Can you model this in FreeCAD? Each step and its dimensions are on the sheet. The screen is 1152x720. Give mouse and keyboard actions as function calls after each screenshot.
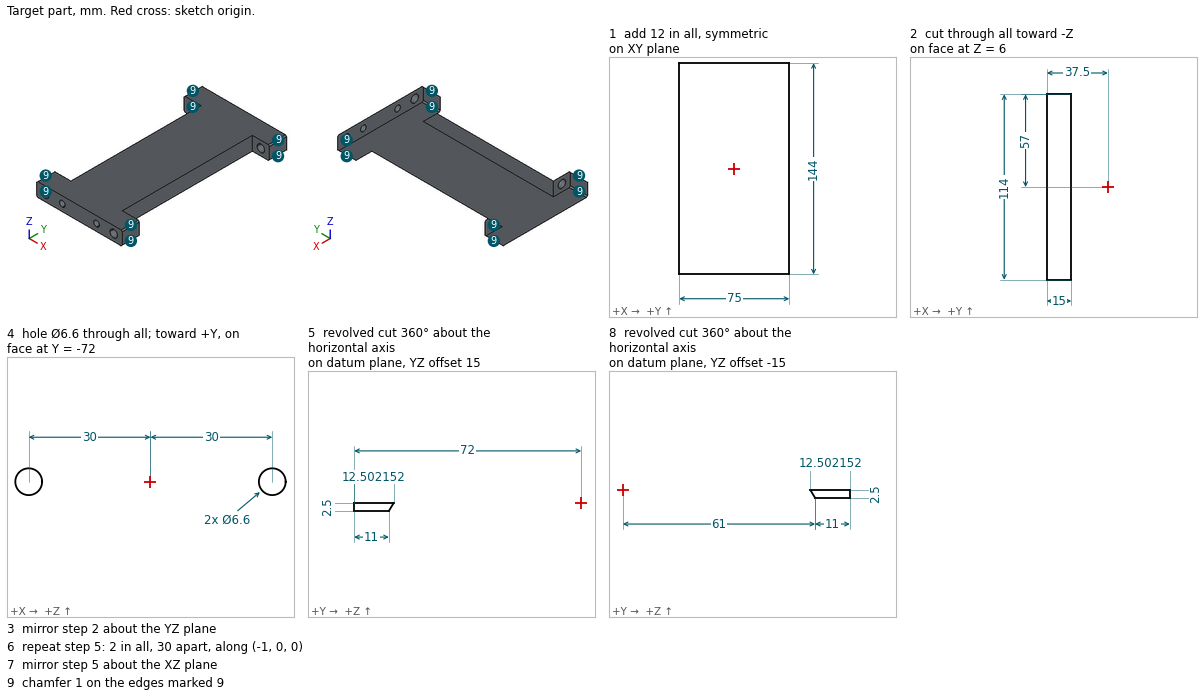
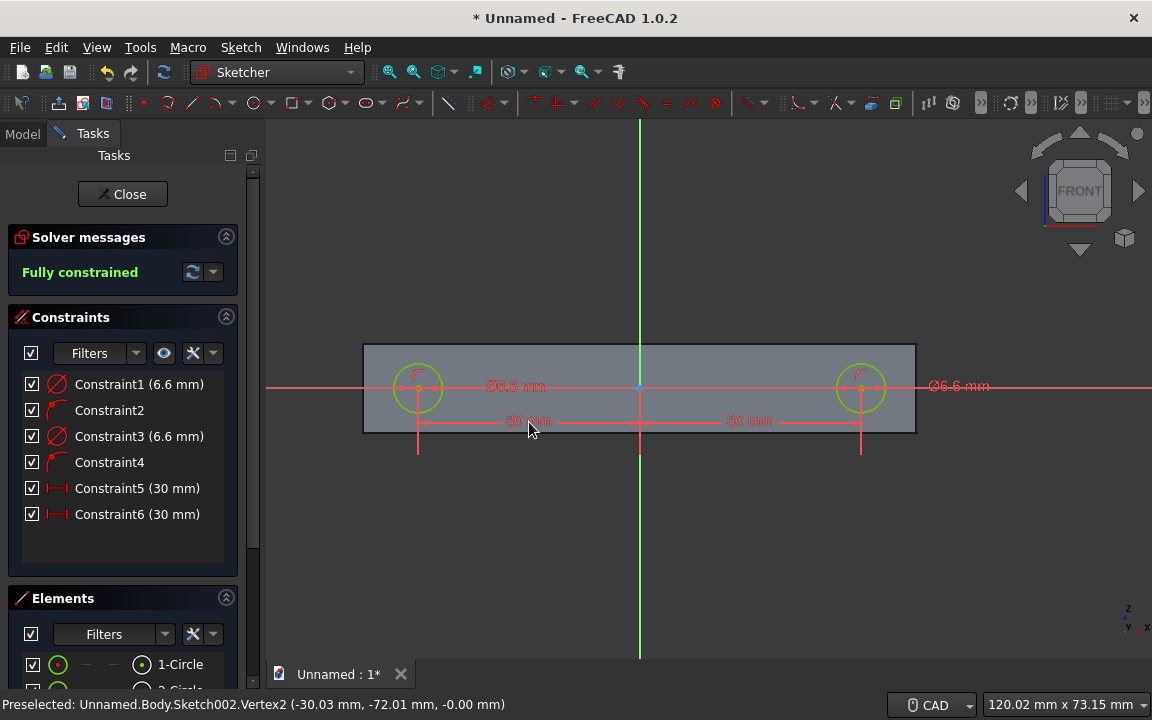
click(123, 194)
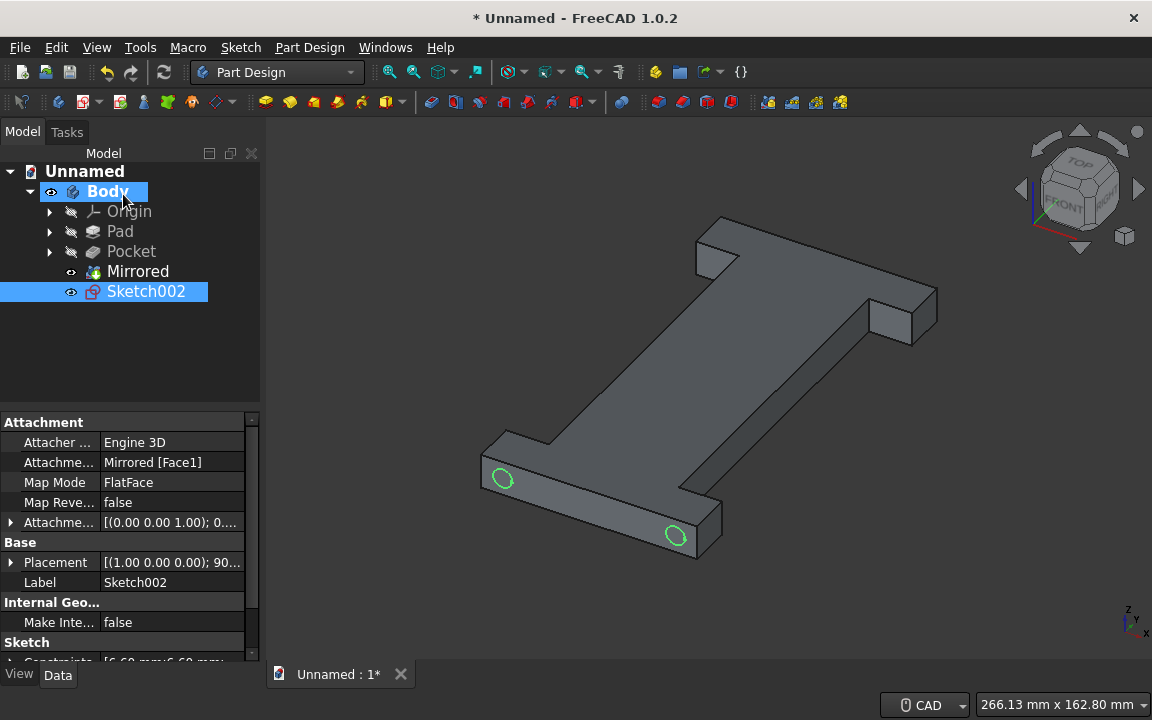
click(456, 102)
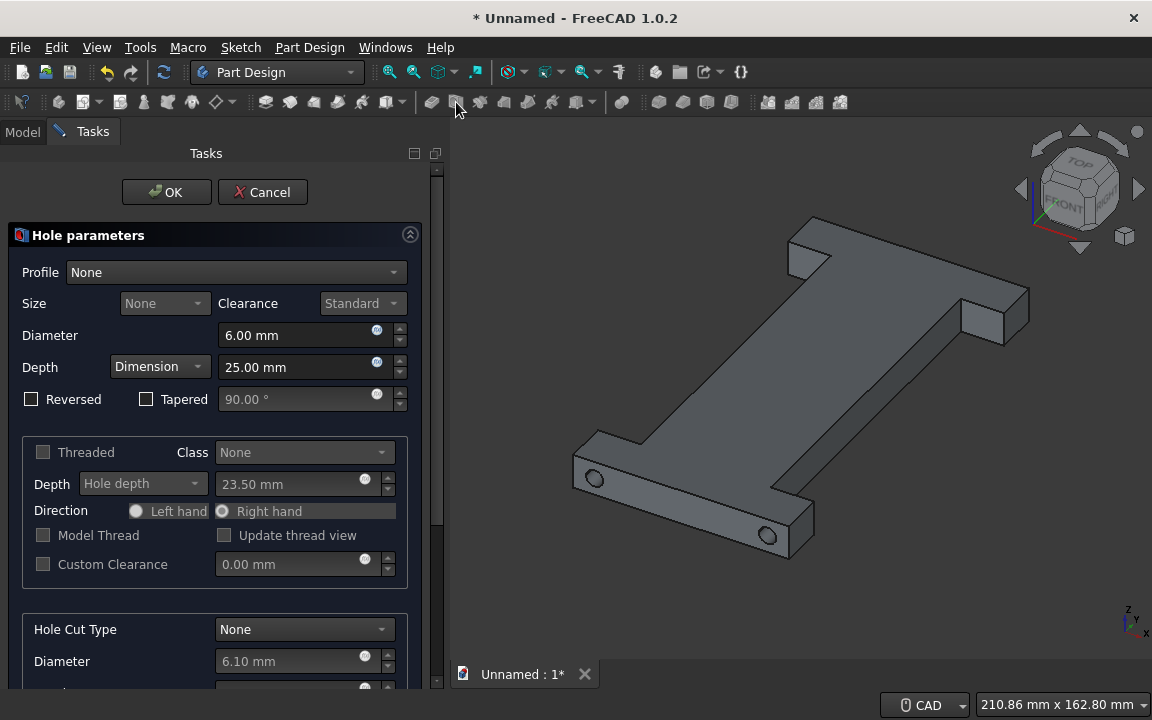
triple_click(305, 335)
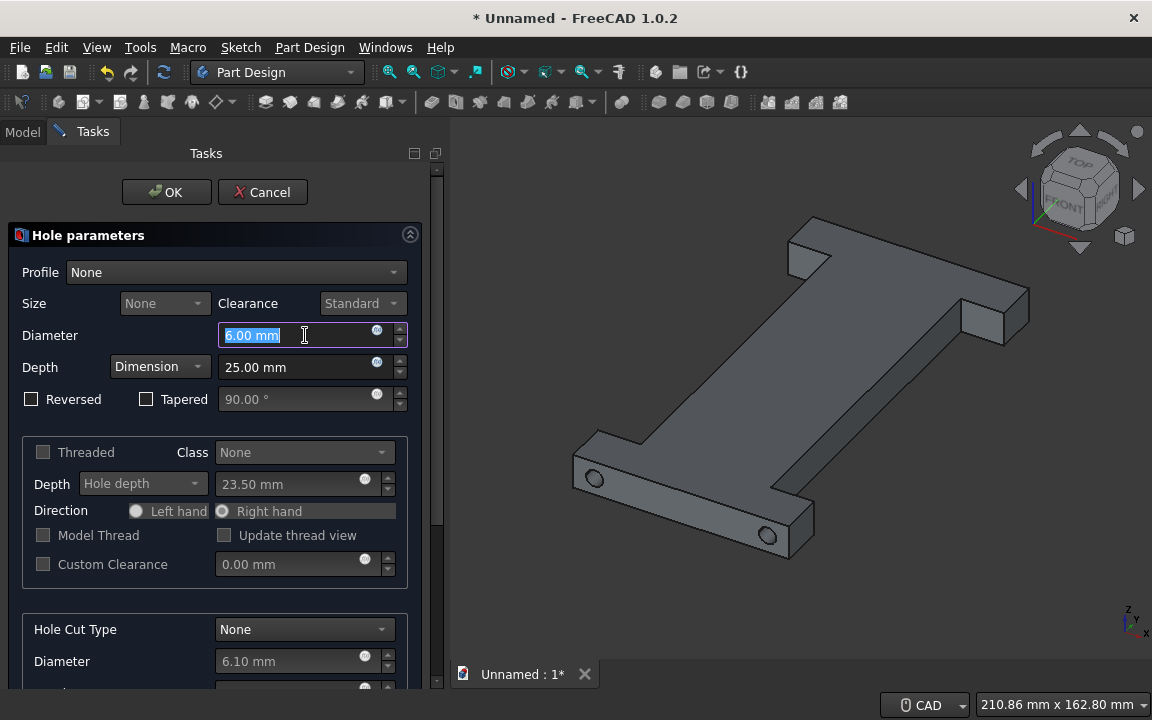
text(6.6)
key(Tab)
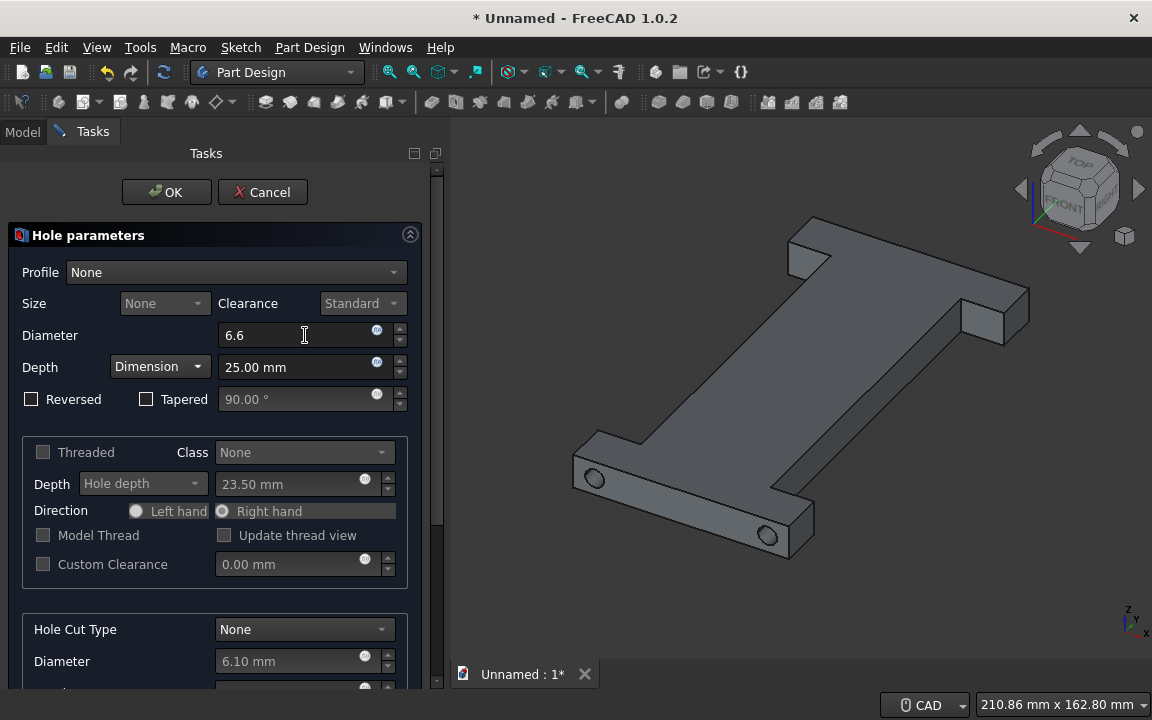
click(161, 366)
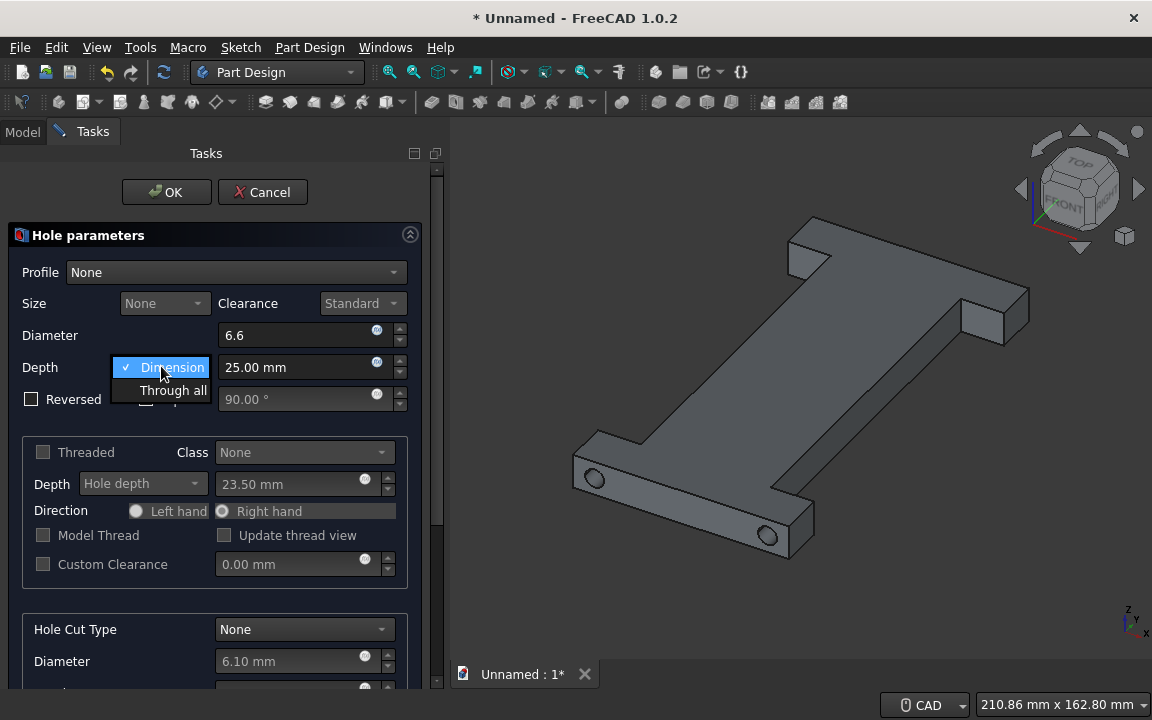
click(160, 390)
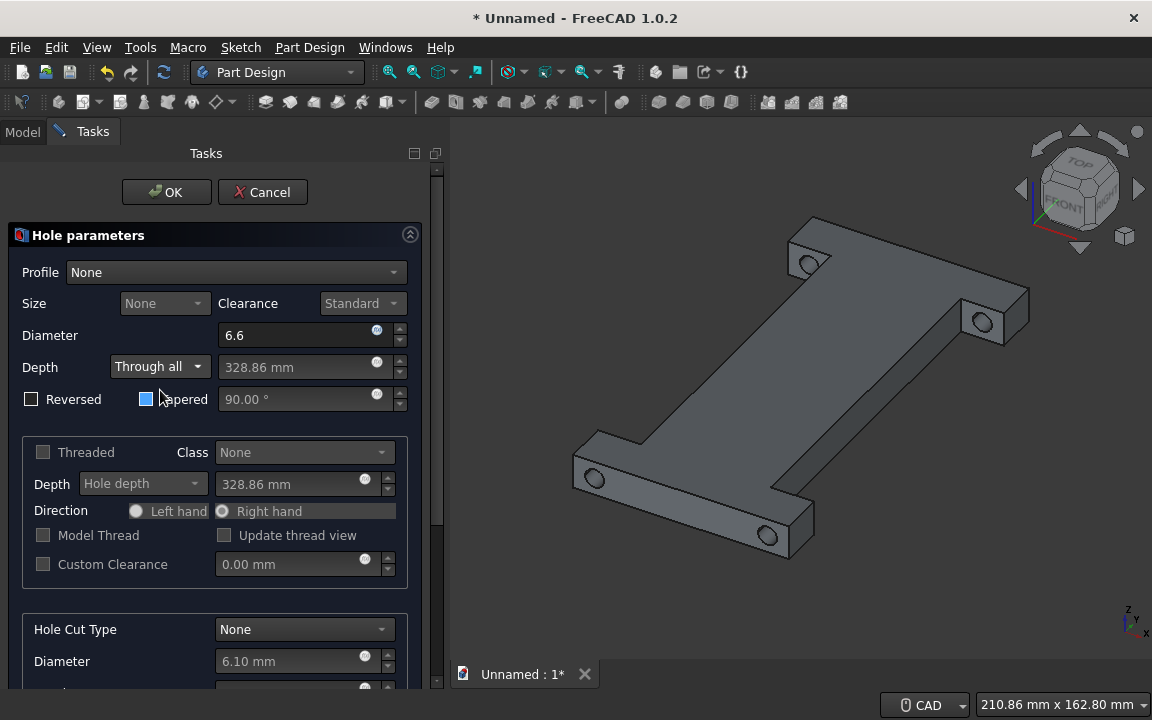
click(167, 192)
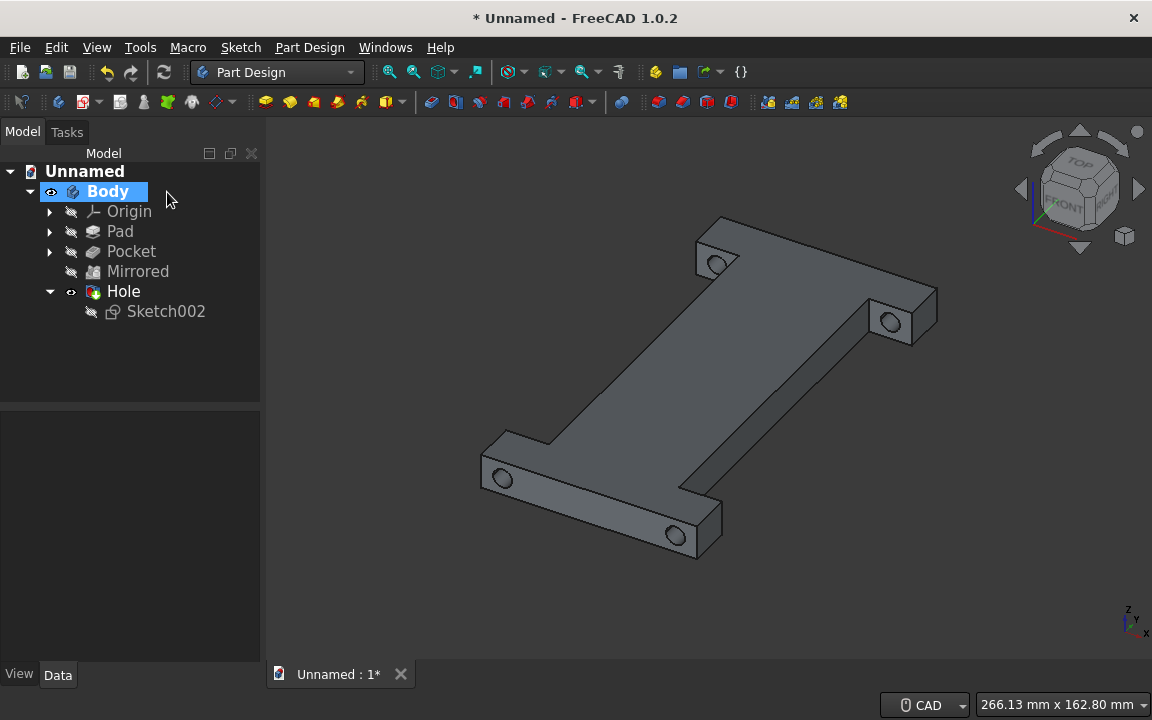
click(50, 212)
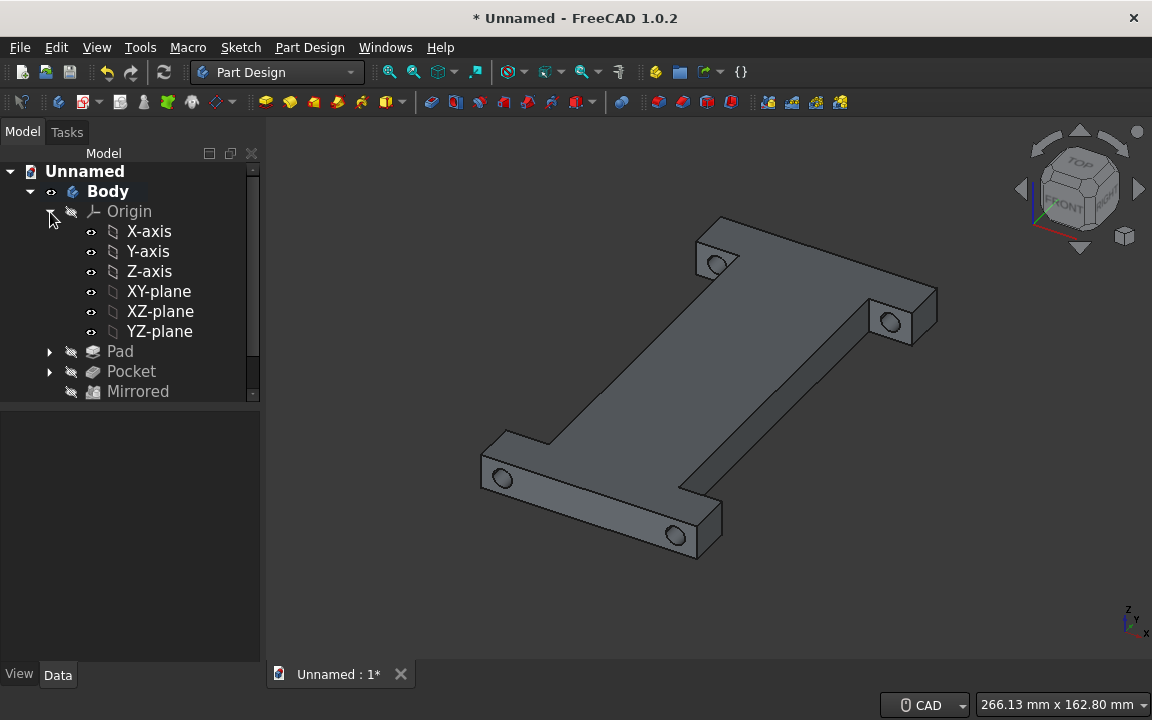
click(136, 332)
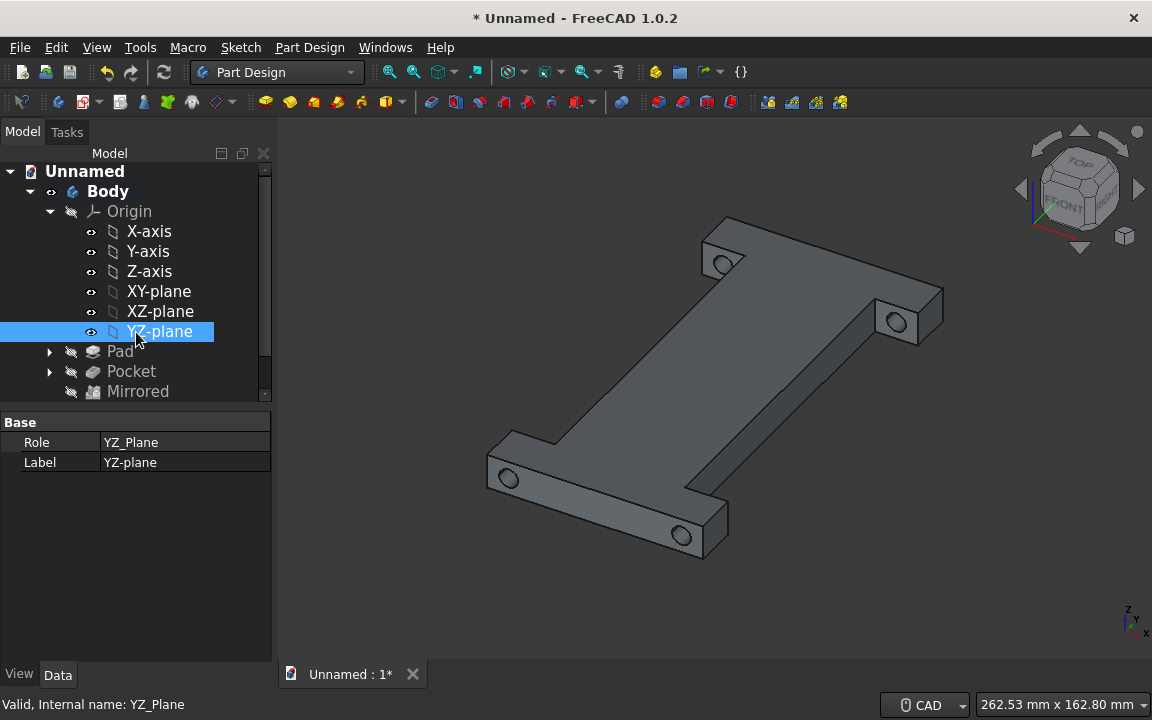
click(216, 102)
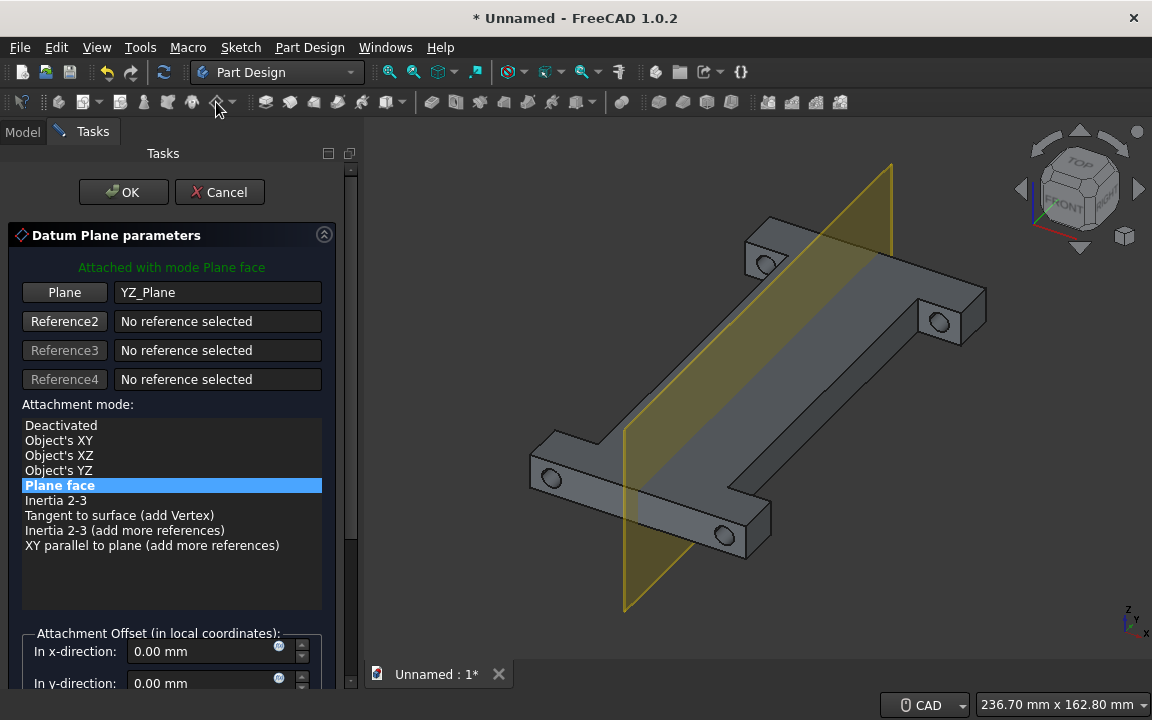
scroll(351, 426, down, 2)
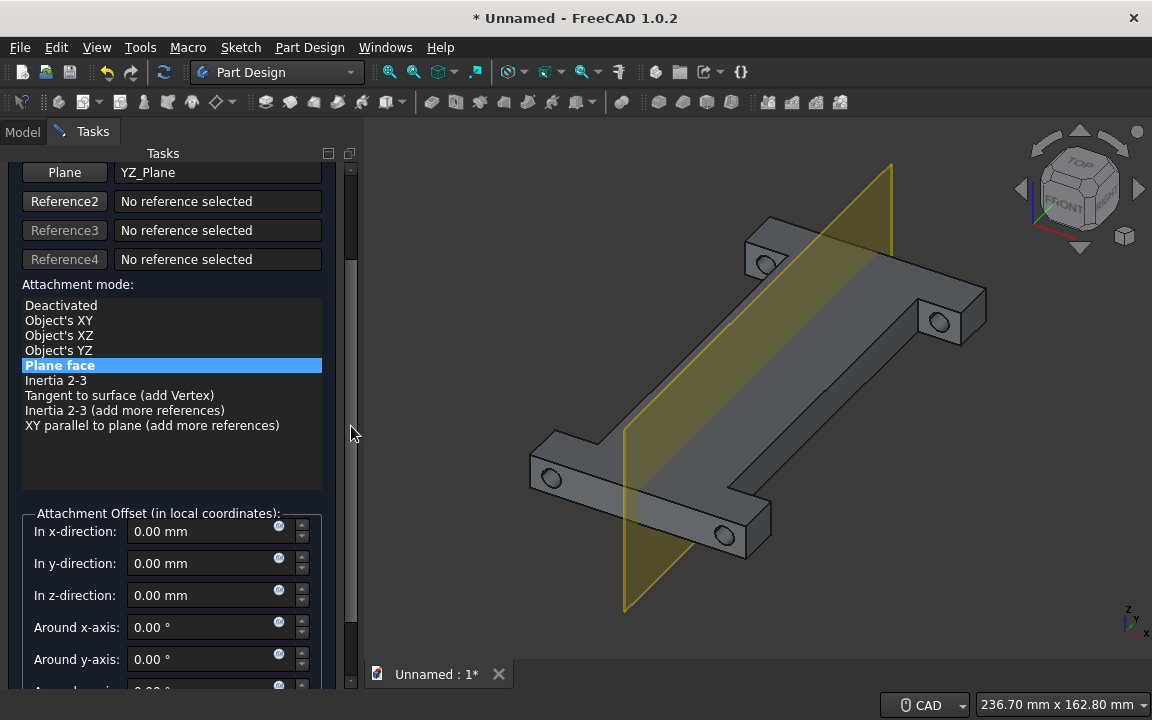
triple_click(210, 595)